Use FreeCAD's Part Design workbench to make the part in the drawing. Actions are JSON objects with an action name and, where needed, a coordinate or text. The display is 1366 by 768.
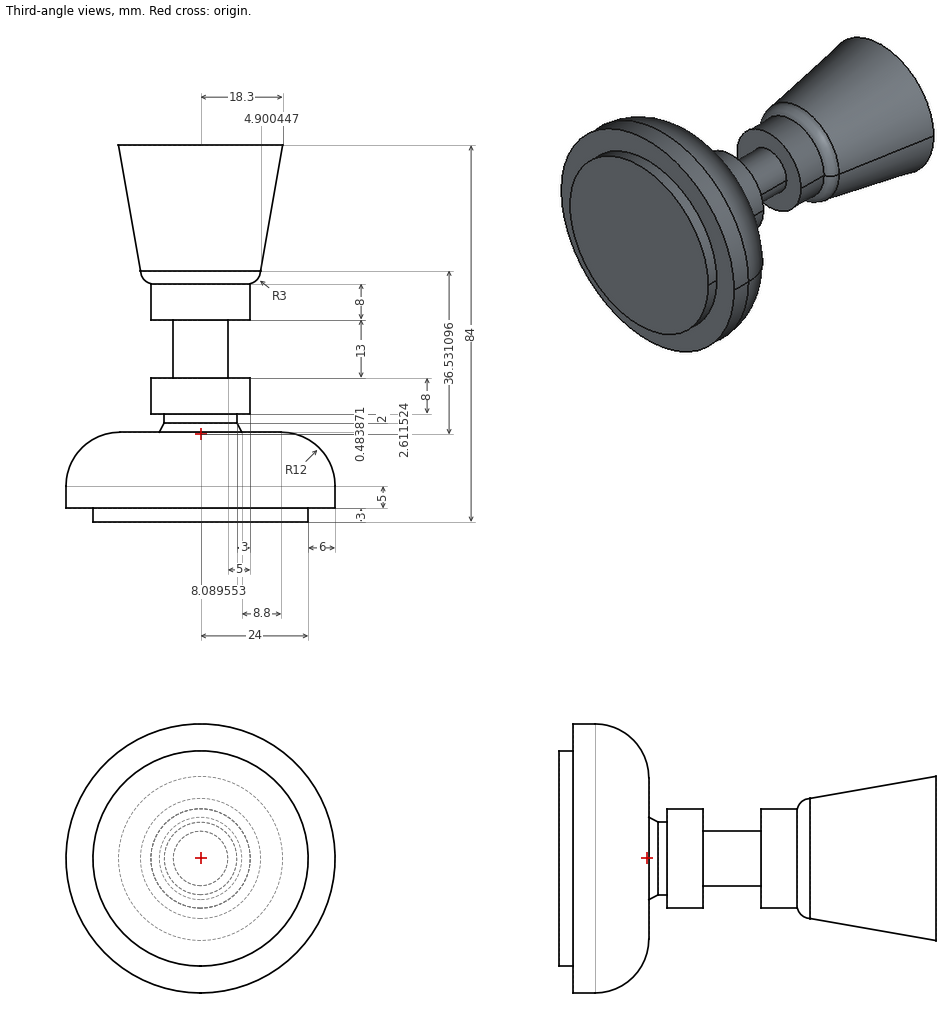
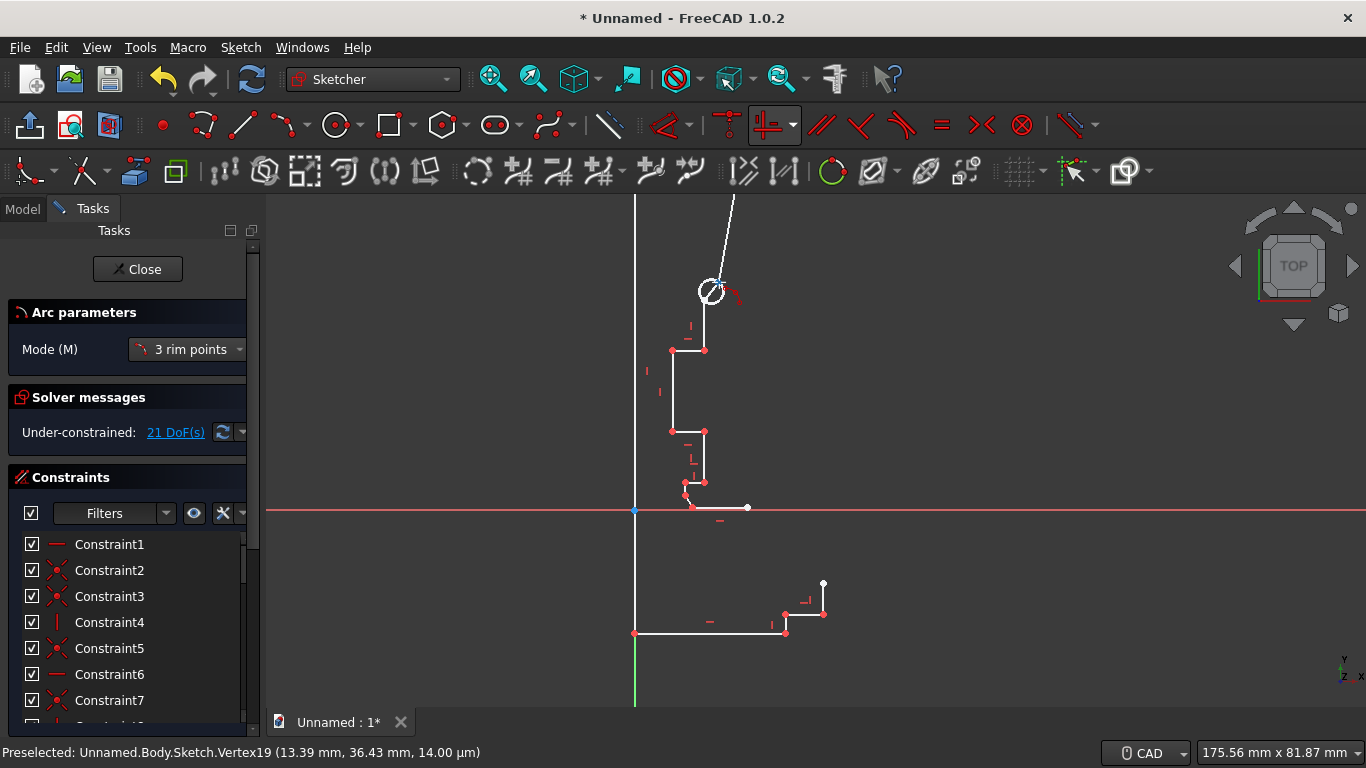
{"action": "scroll", "coordinate": [715, 293], "scroll_direction": "up", "scroll_amount": 7}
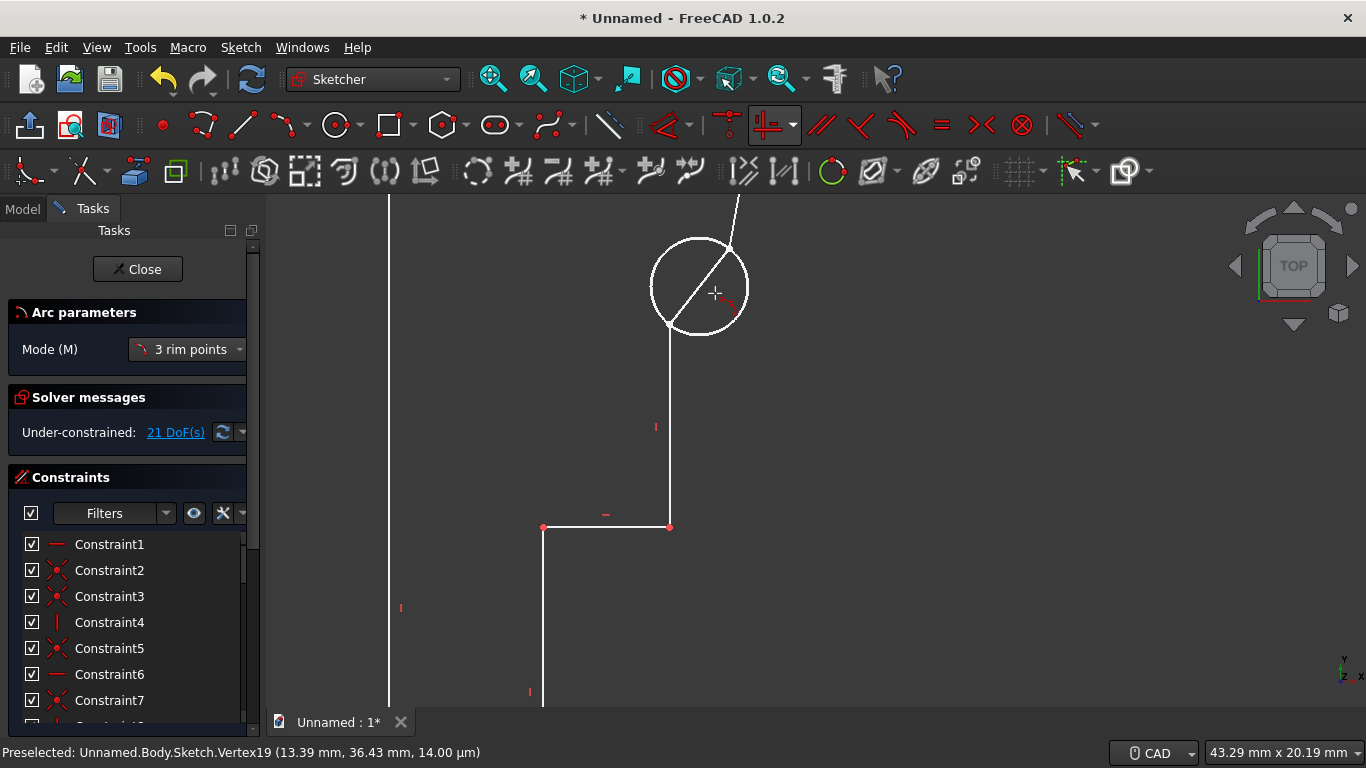
{"action": "left_click", "coordinate": [713, 293]}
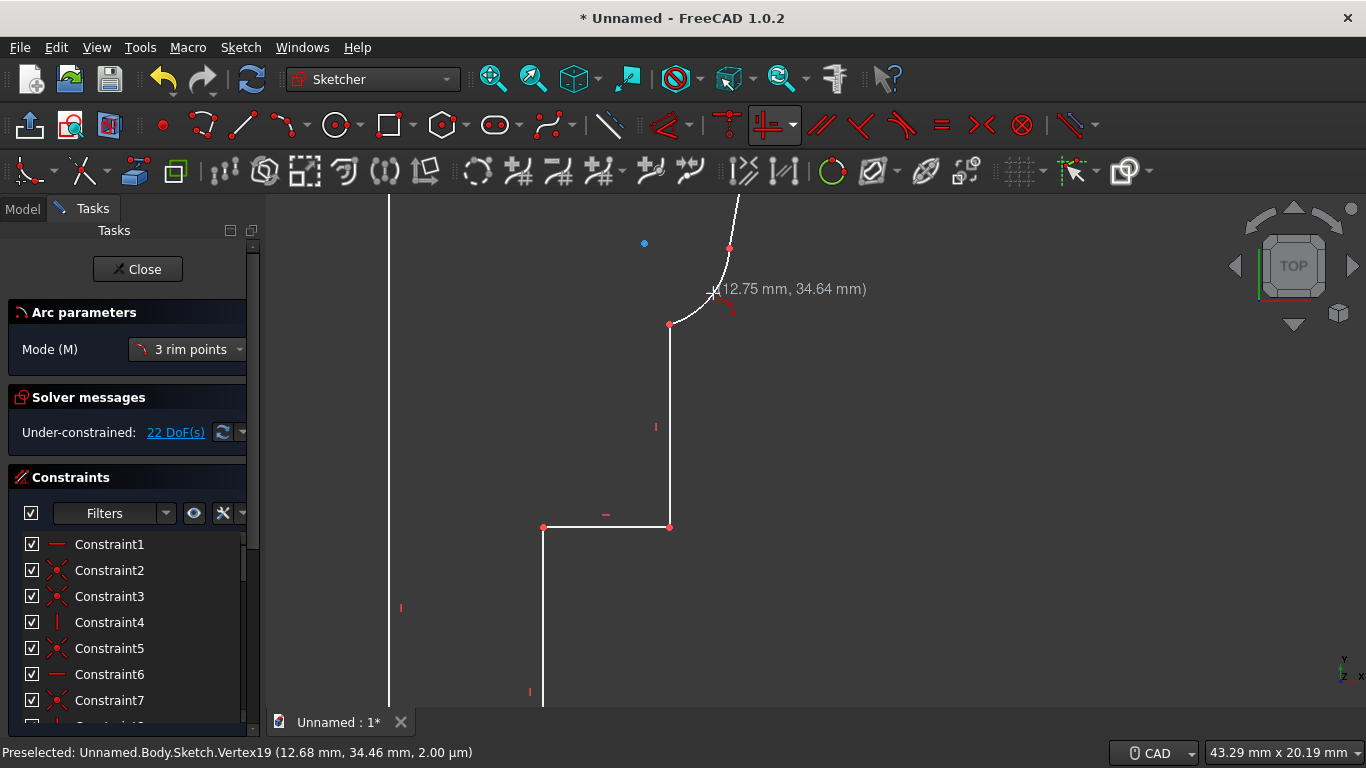
{"action": "scroll", "coordinate": [743, 420], "scroll_direction": "down", "scroll_amount": 9}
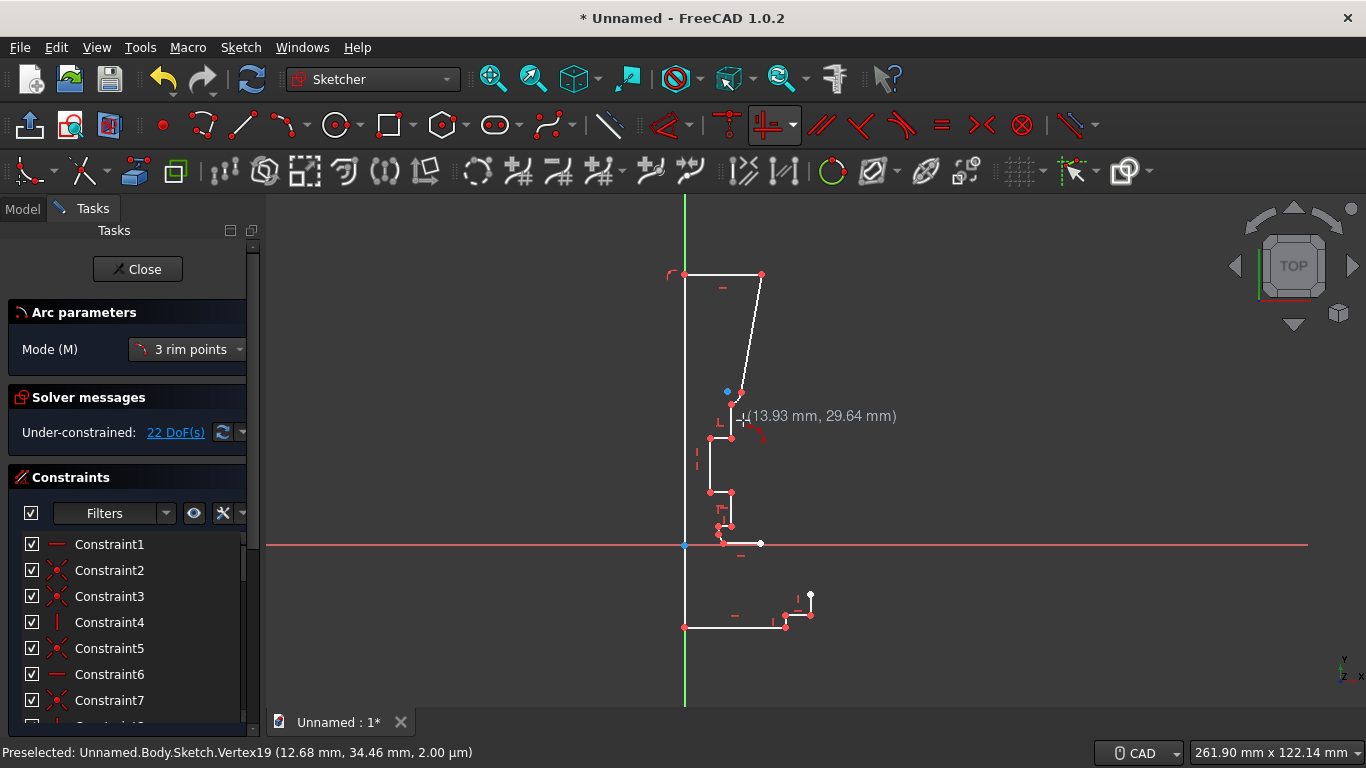
{"action": "scroll", "coordinate": [811, 593], "scroll_direction": "up", "scroll_amount": 3}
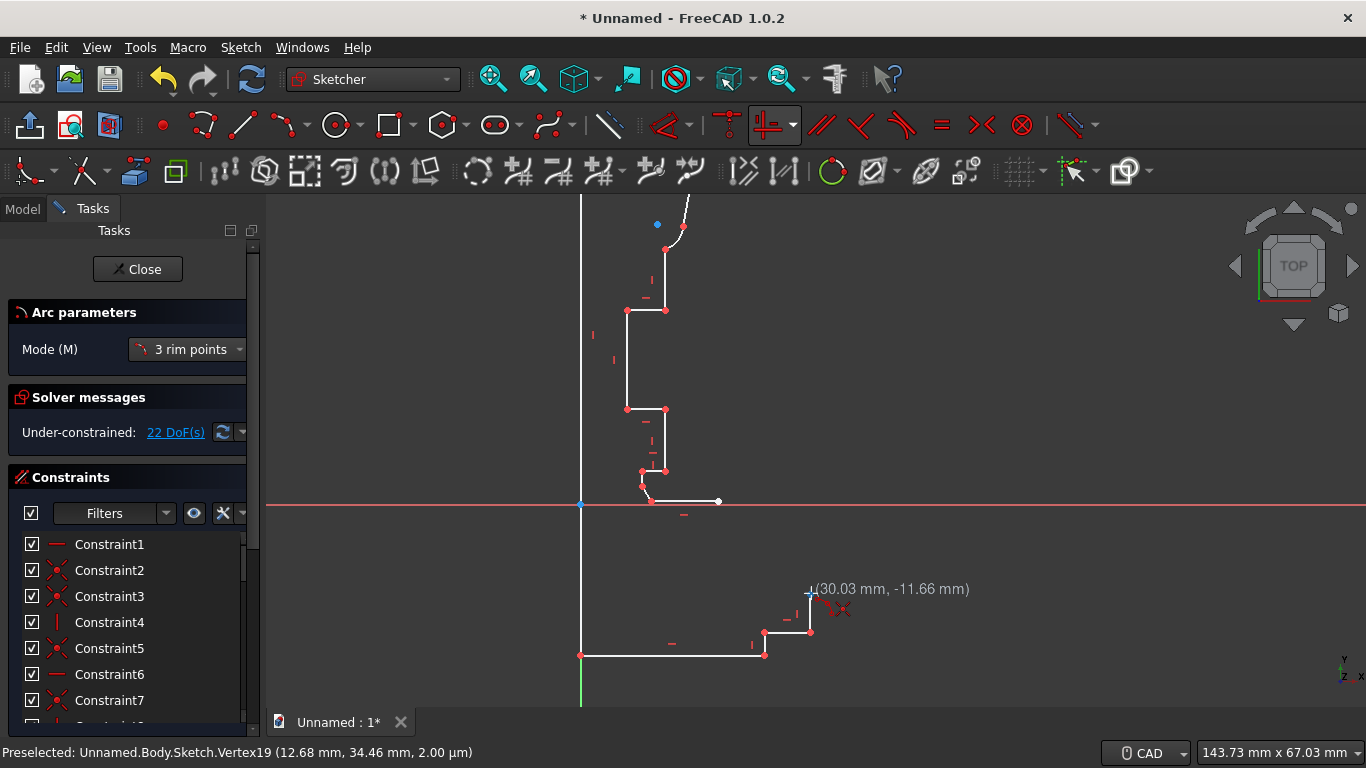
{"action": "left_click", "coordinate": [810, 595]}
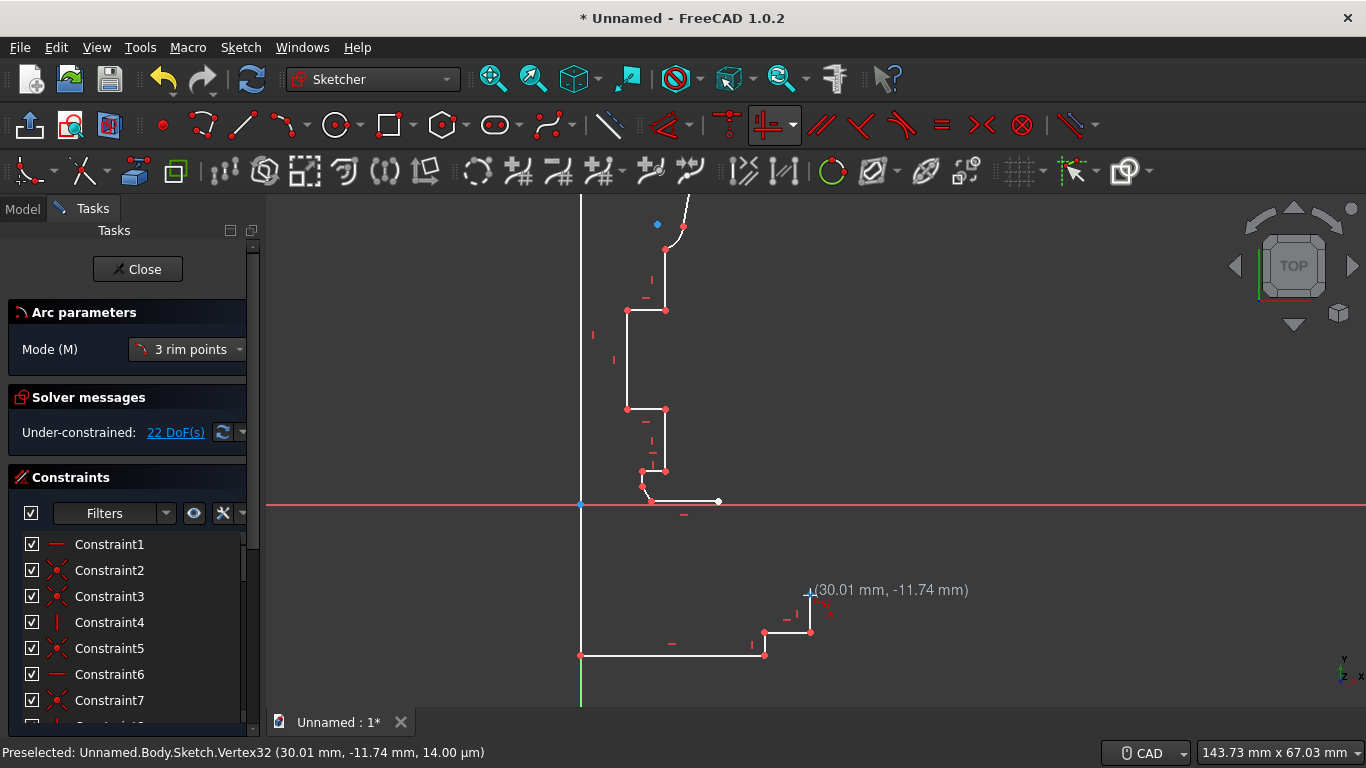
{"action": "scroll", "coordinate": [719, 501], "scroll_direction": "up", "scroll_amount": 8}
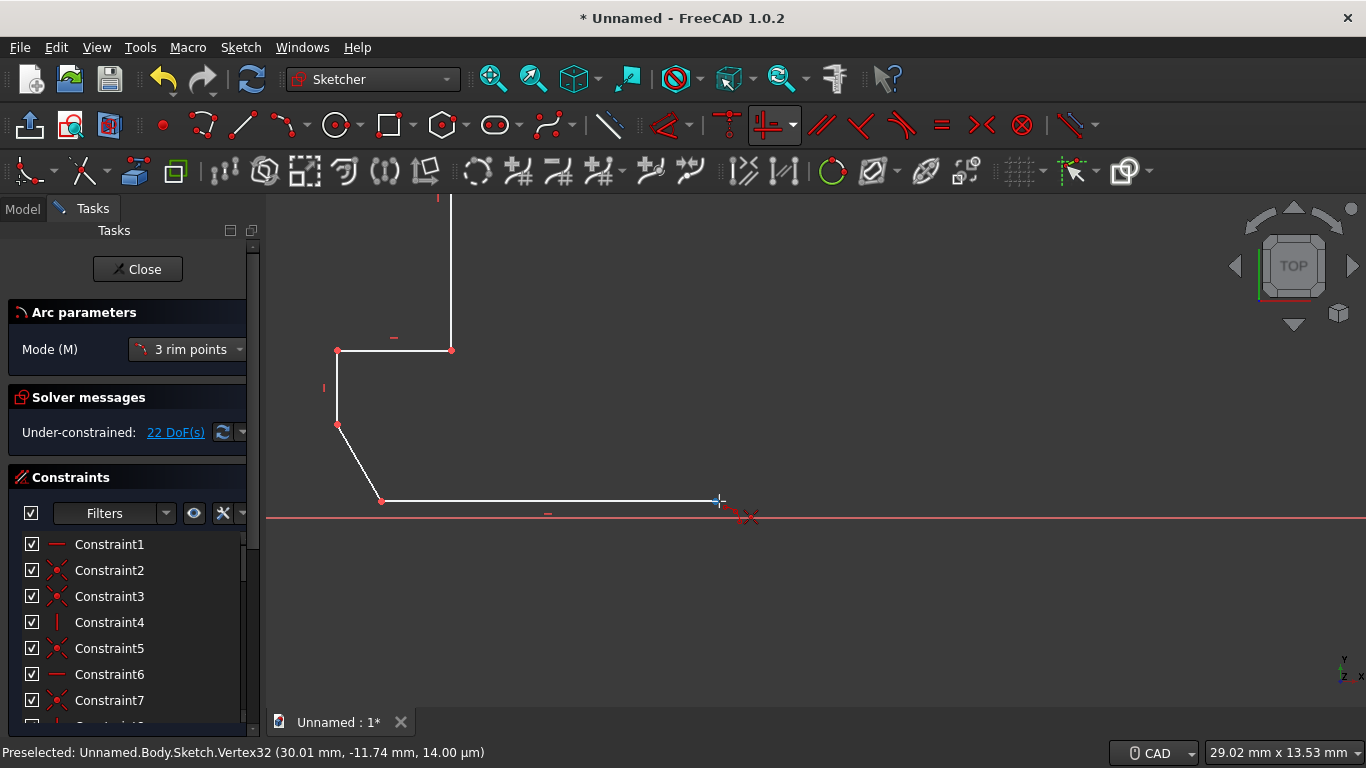
{"action": "left_click", "coordinate": [715, 501]}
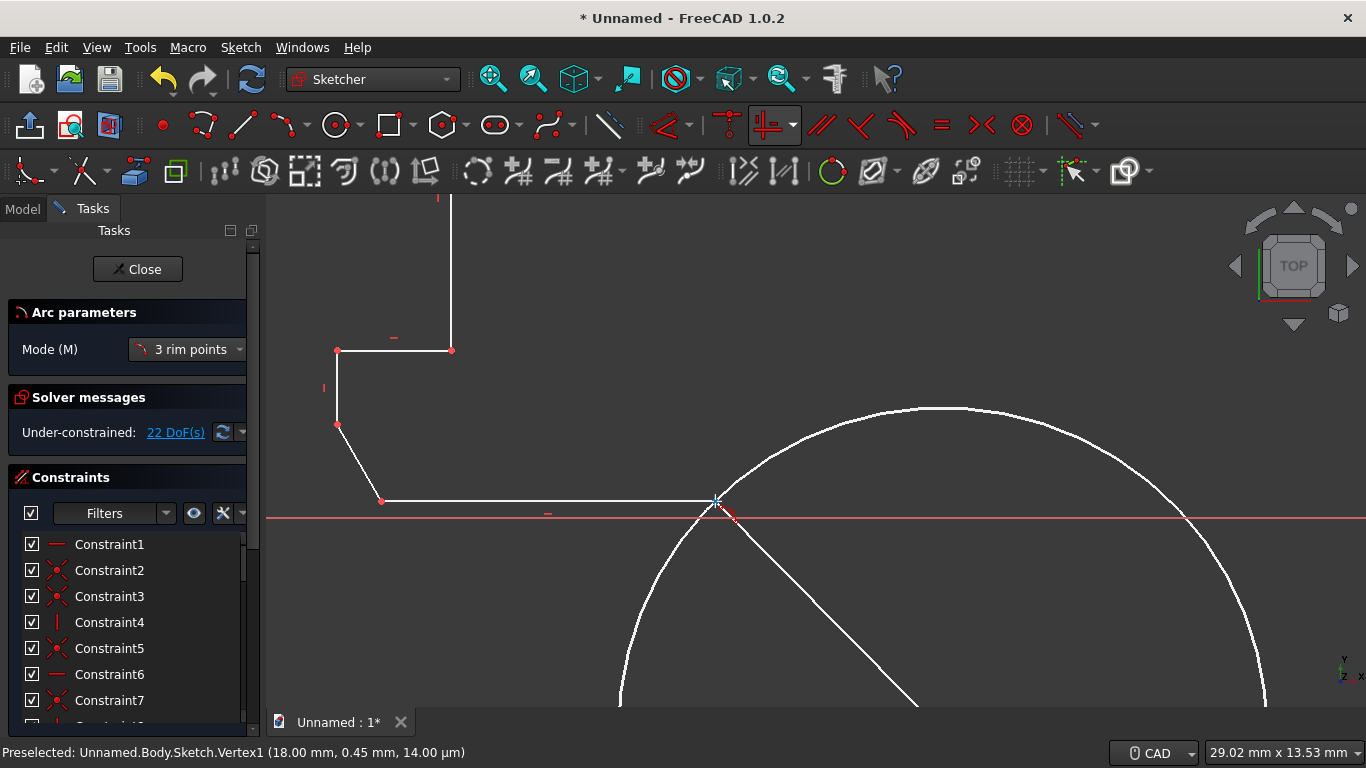
{"action": "scroll", "coordinate": [766, 548], "scroll_direction": "down", "scroll_amount": 11}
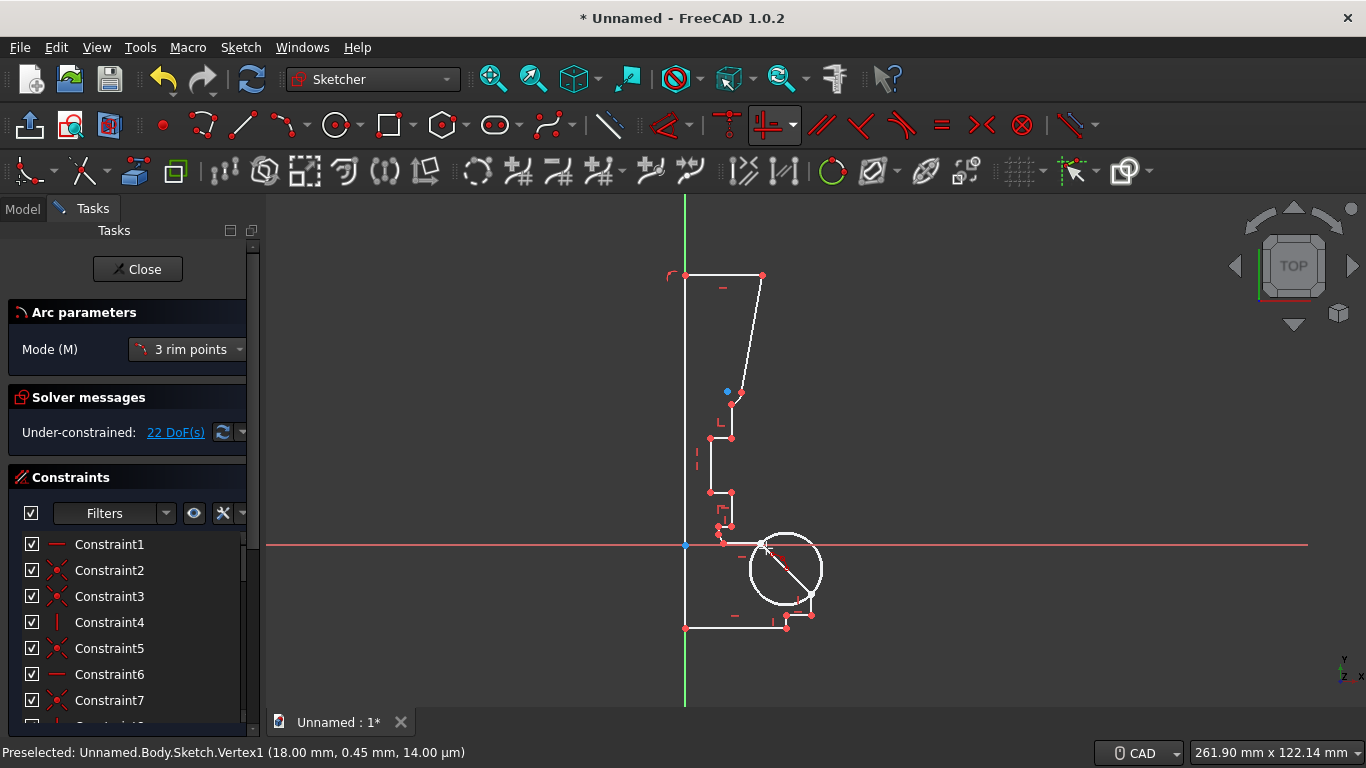
{"action": "left_click", "coordinate": [802, 564]}
{"action": "key", "text": "Escape"}